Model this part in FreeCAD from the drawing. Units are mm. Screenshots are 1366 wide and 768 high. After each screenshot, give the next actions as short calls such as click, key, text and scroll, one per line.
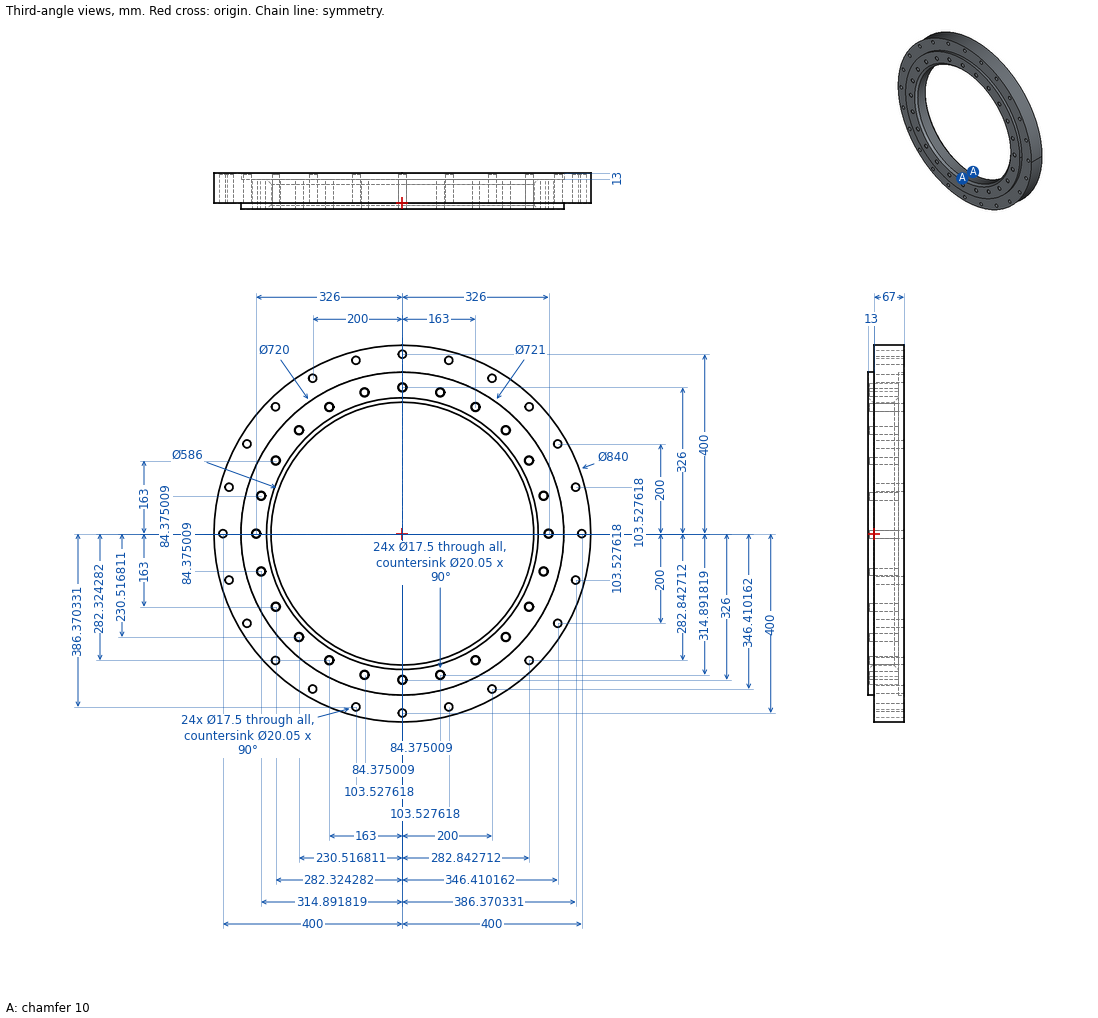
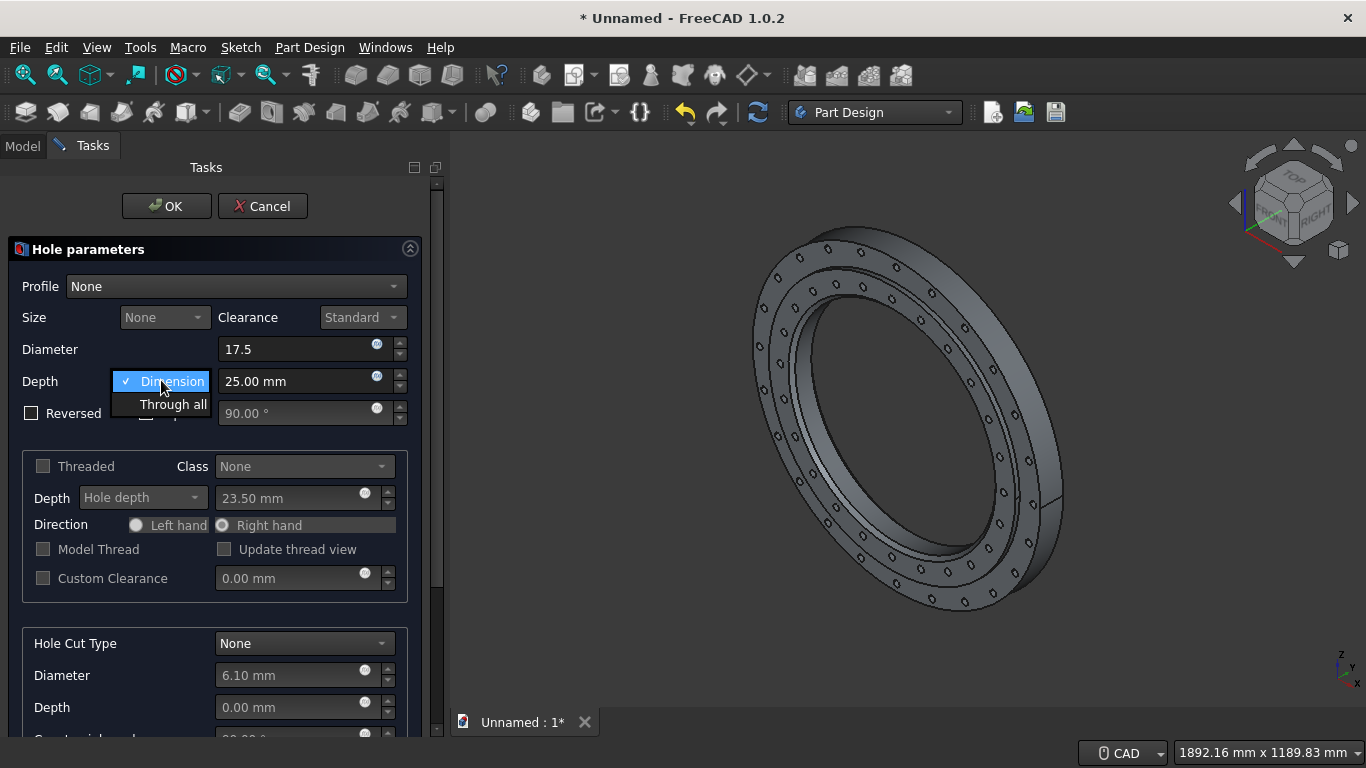
click(160, 404)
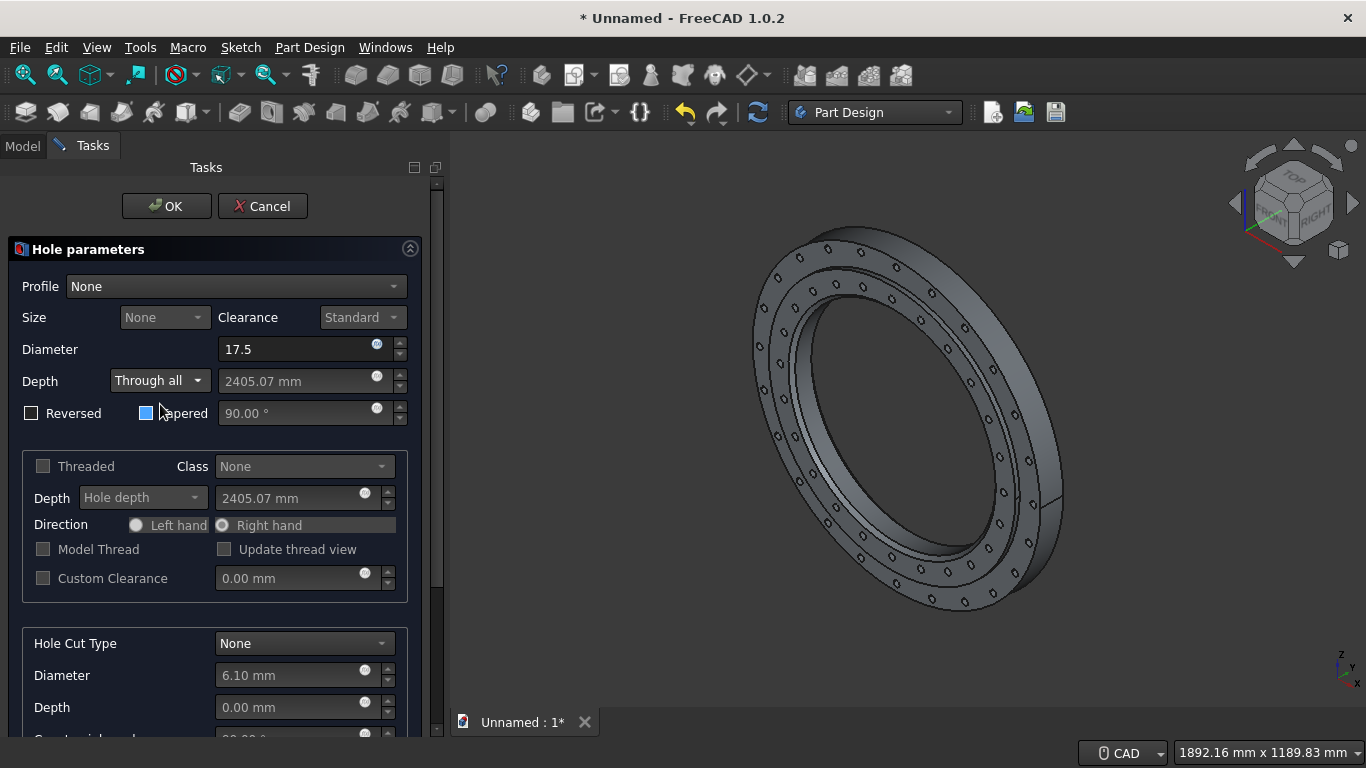
click(306, 644)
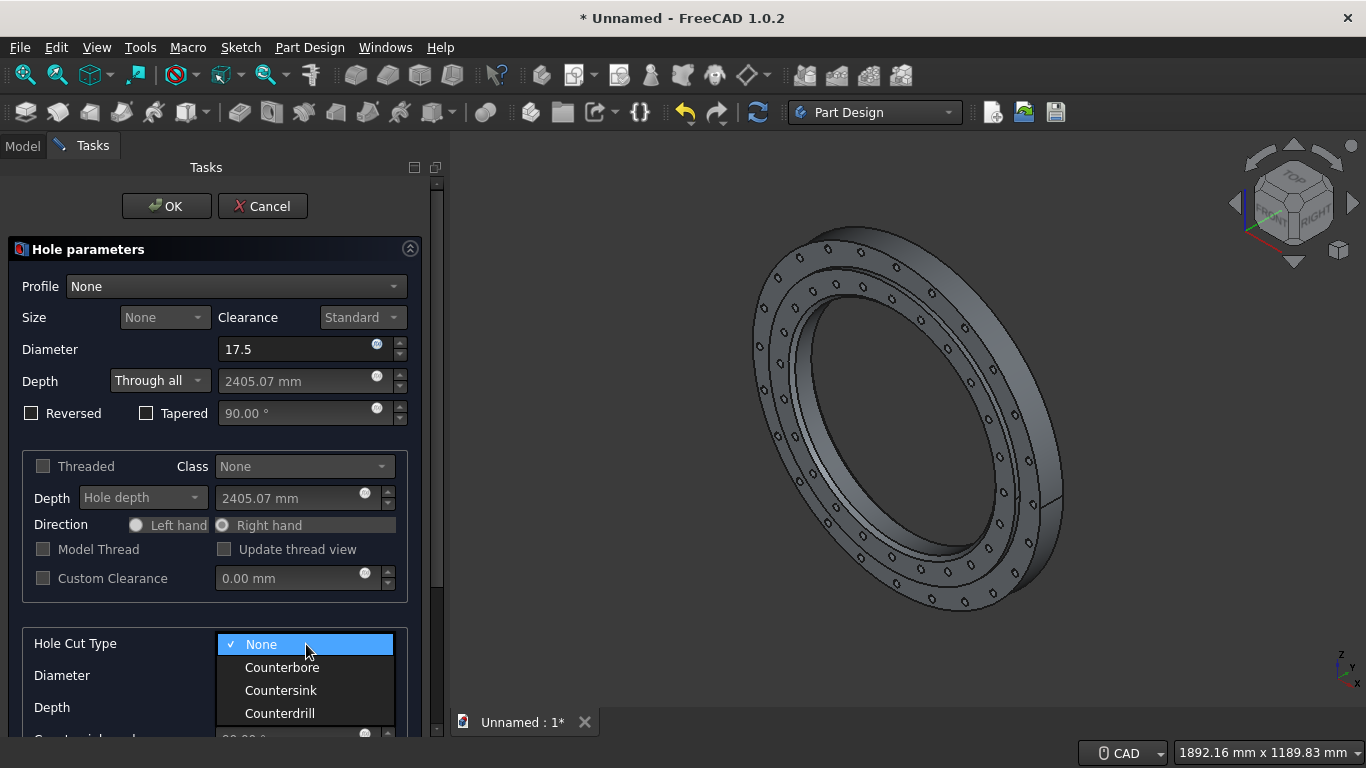
click(304, 690)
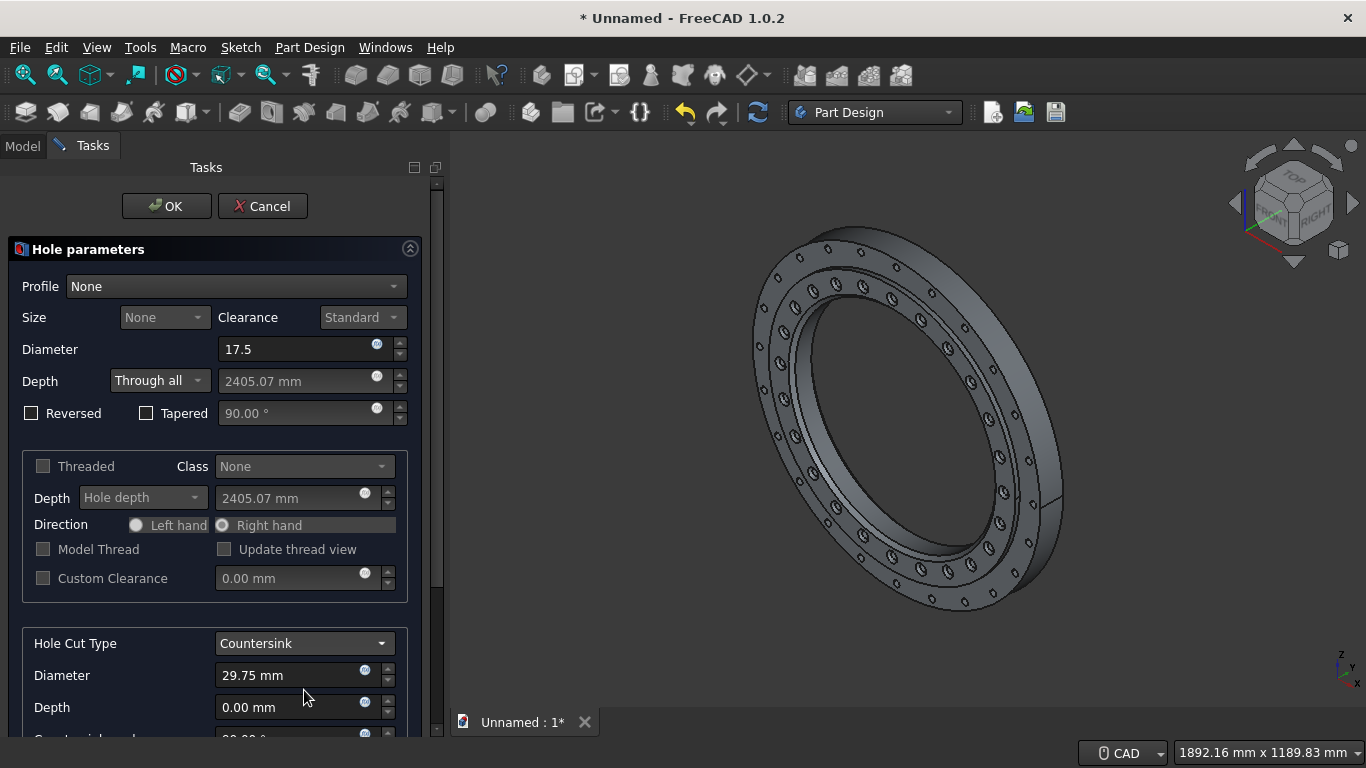
triple_click(298, 675)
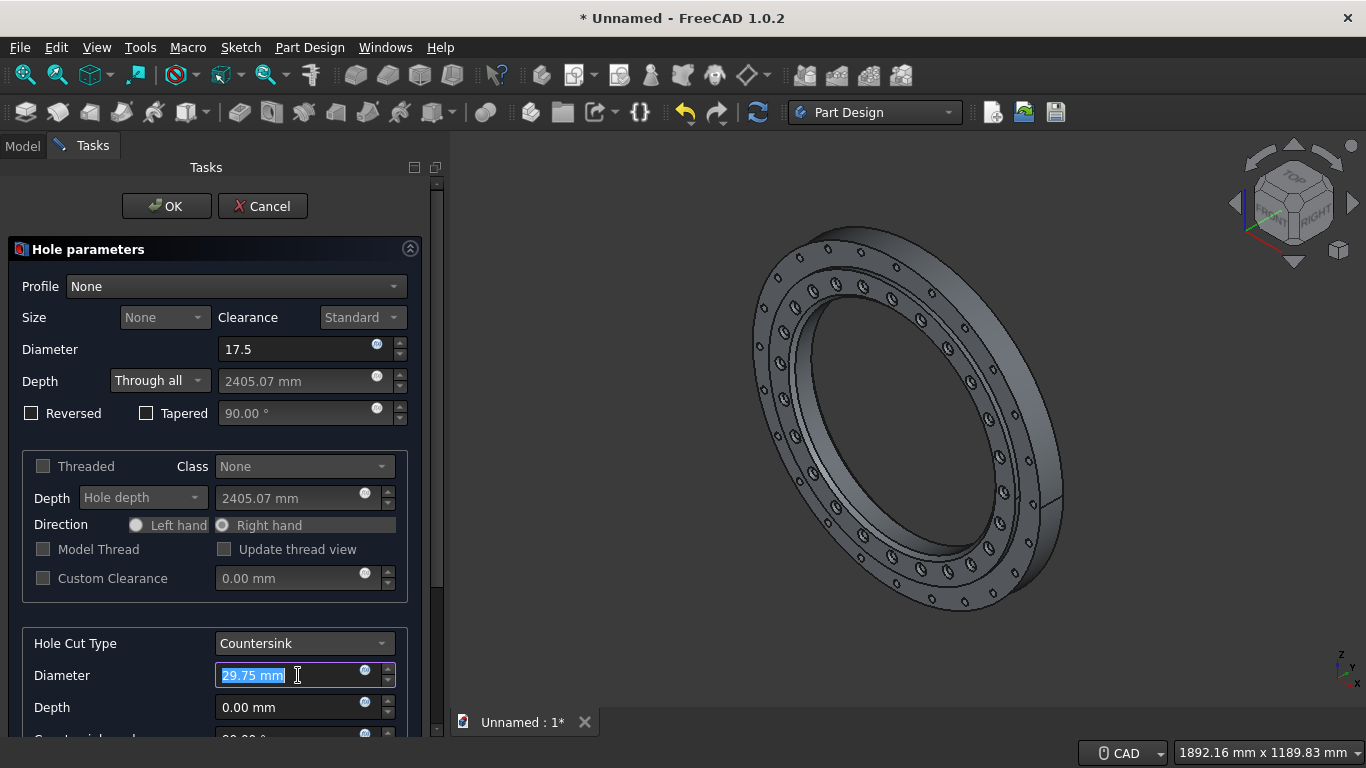
text(20.05)
key(Tab)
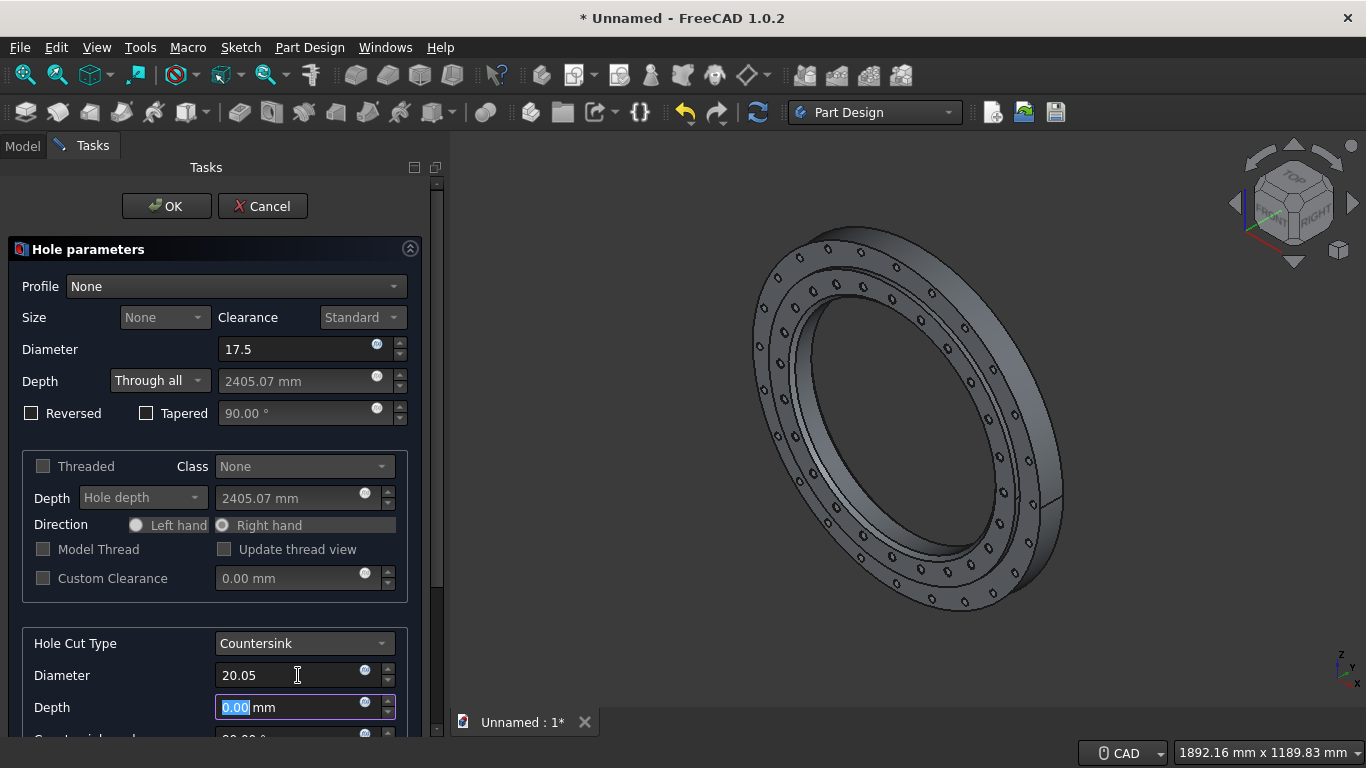
click(167, 206)